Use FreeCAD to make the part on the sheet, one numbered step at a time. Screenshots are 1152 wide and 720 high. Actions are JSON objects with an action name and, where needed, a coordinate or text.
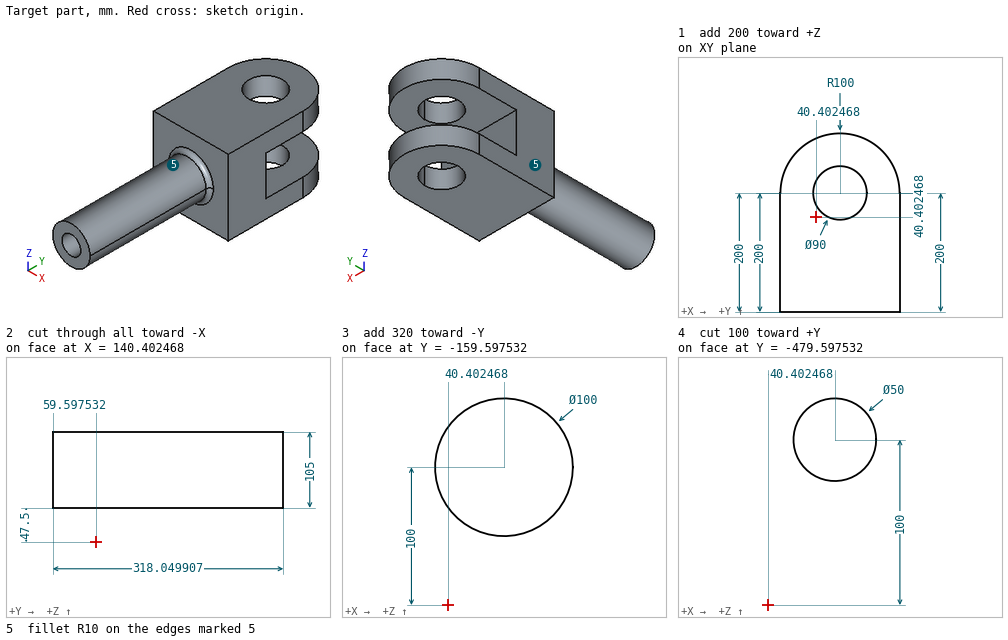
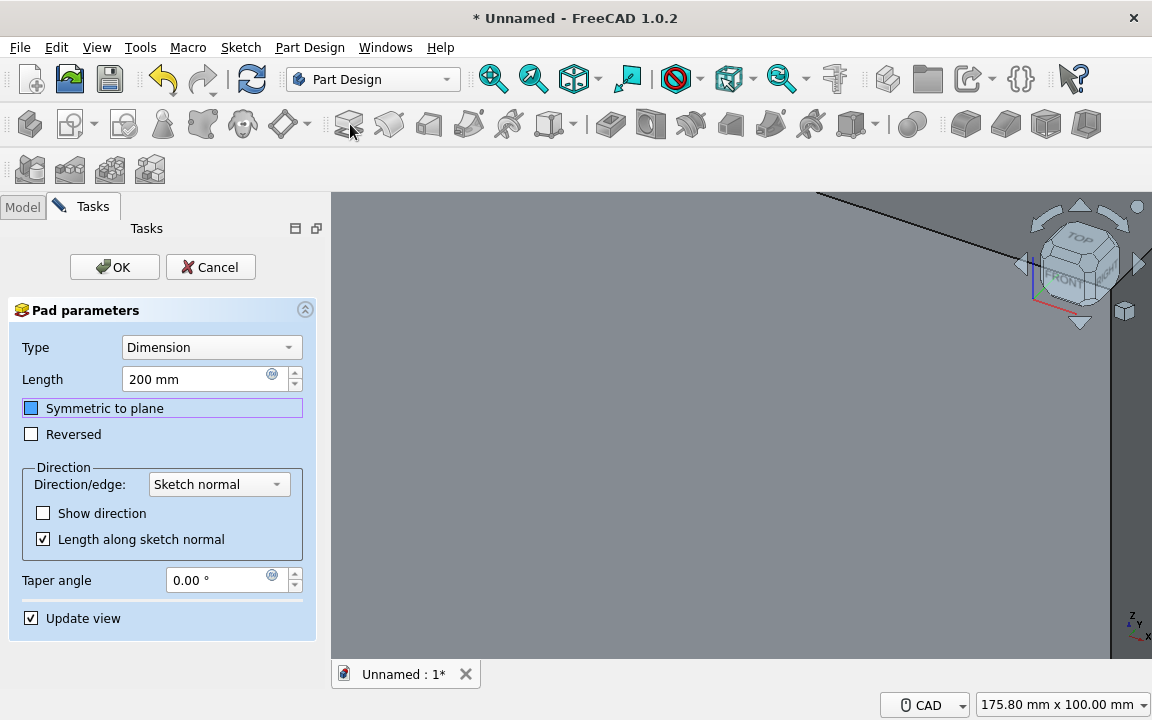
{"action": "left_click", "coordinate": [115, 267]}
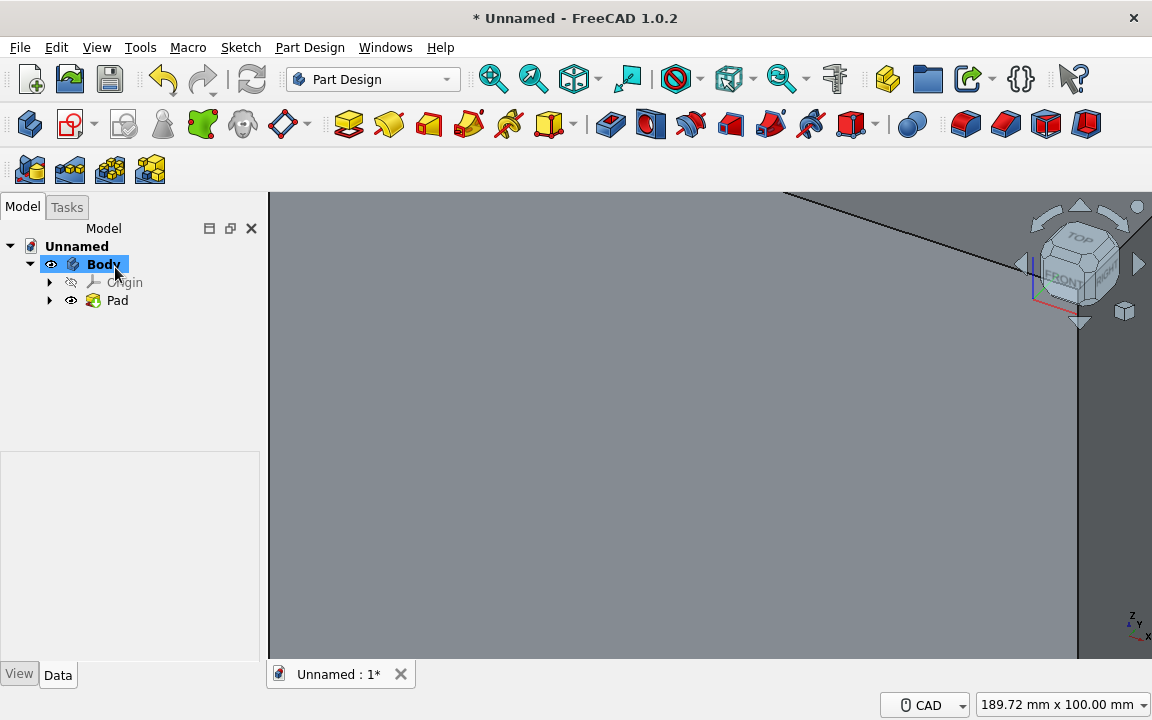
{"action": "key", "text": "v f"}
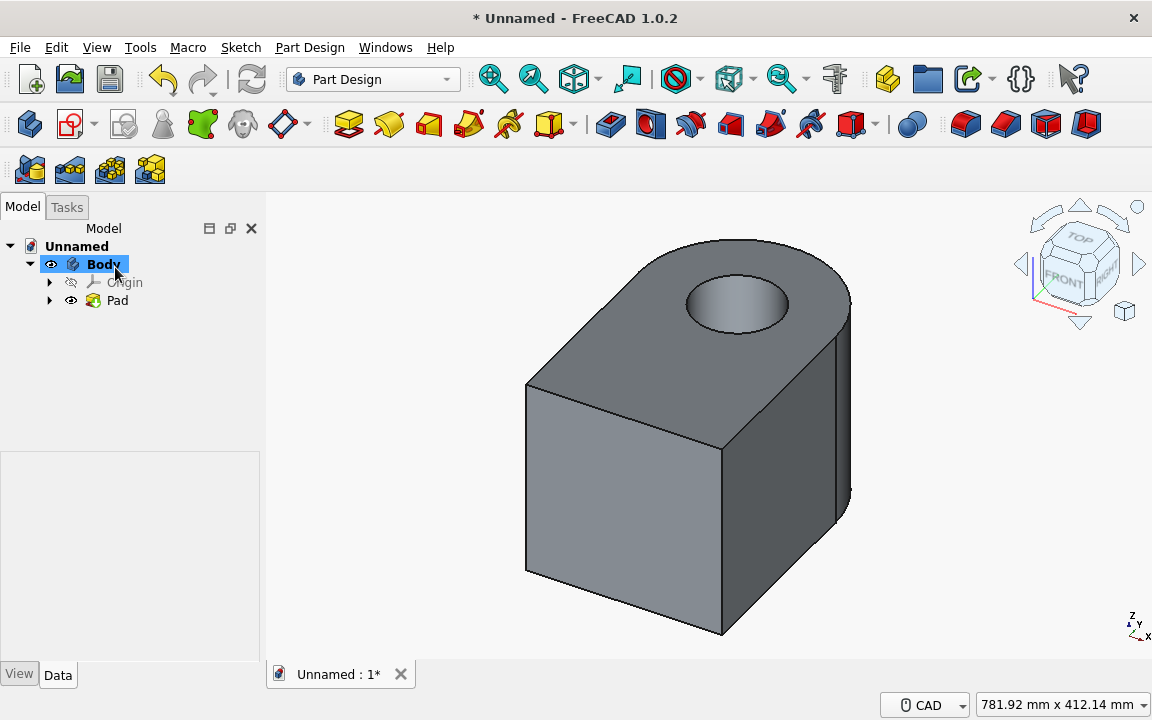
{"action": "left_click", "coordinate": [779, 485]}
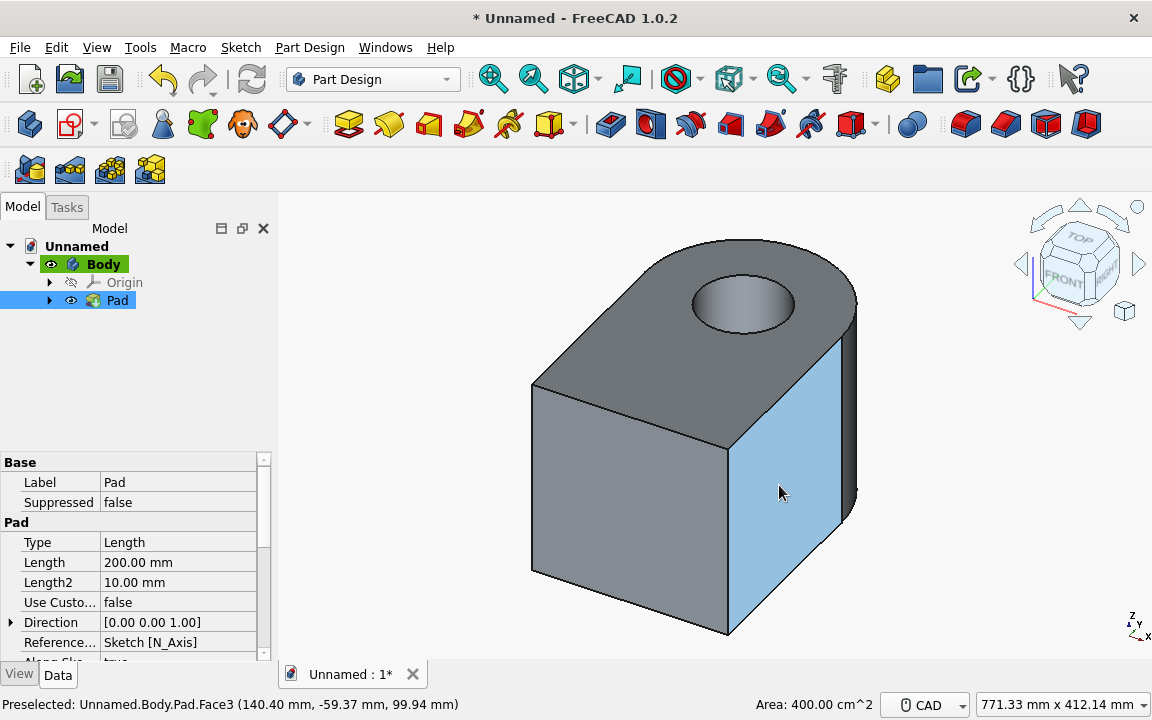
{"action": "left_click", "coordinate": [70, 124]}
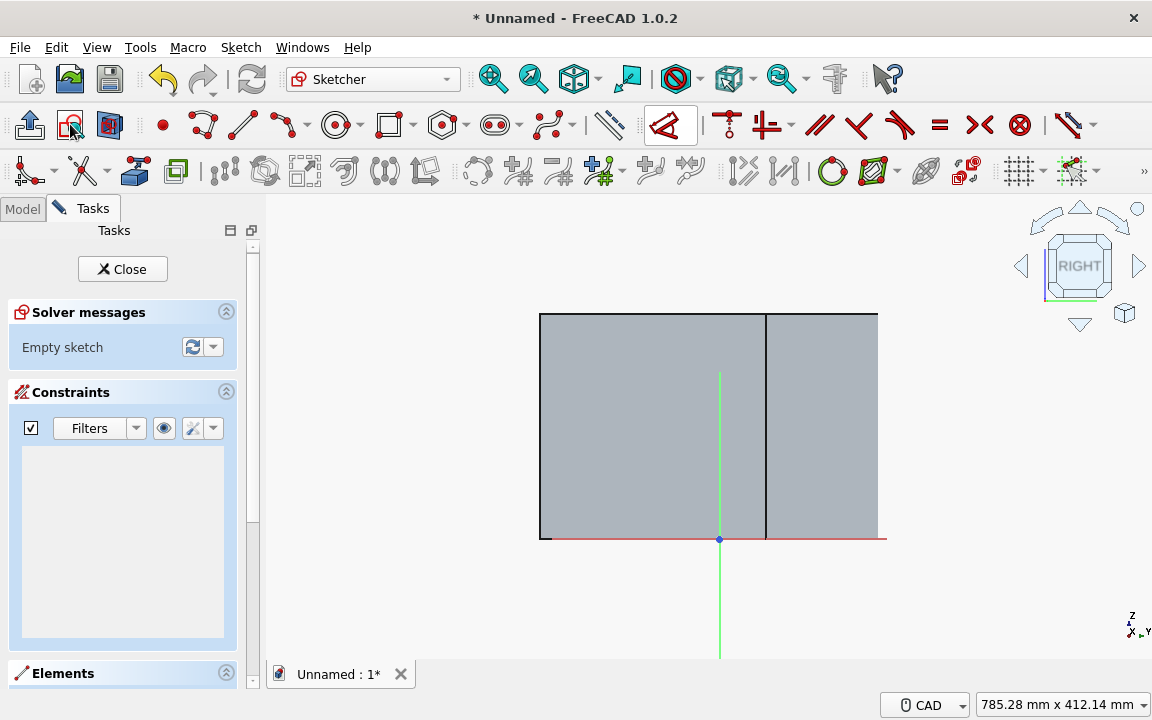
{"action": "scroll", "coordinate": [294, 305], "scroll_direction": "down", "scroll_amount": 1}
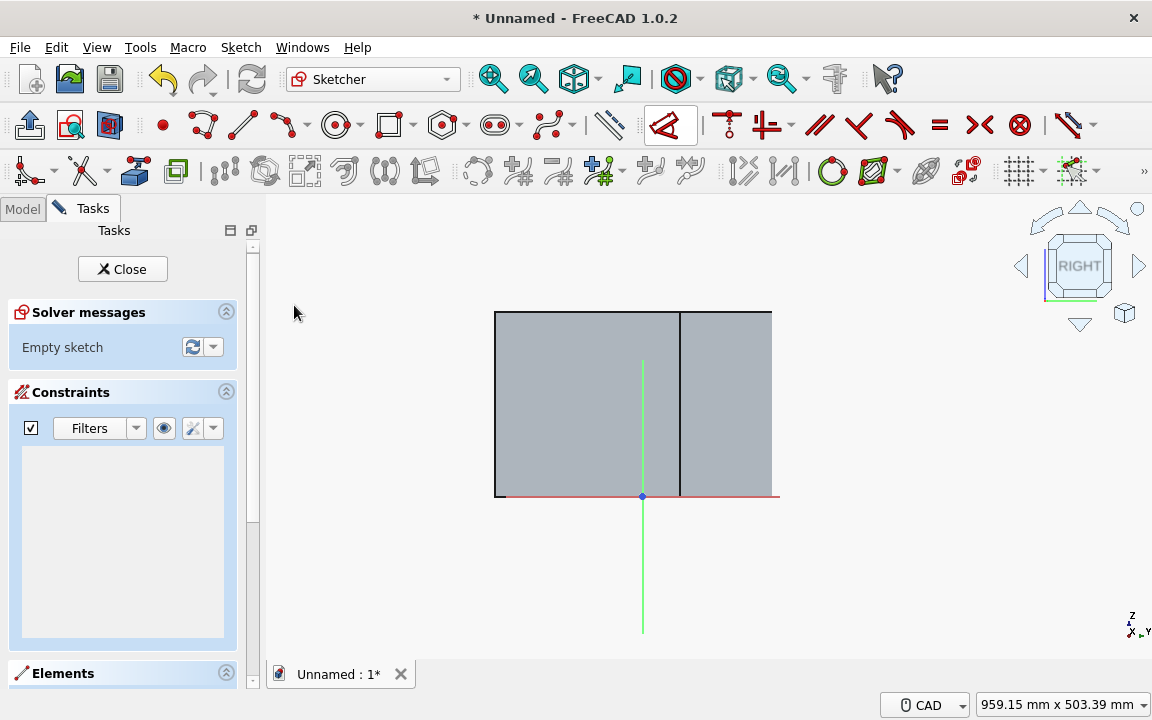
{"action": "scroll", "coordinate": [849, 426], "scroll_direction": "up", "scroll_amount": 3}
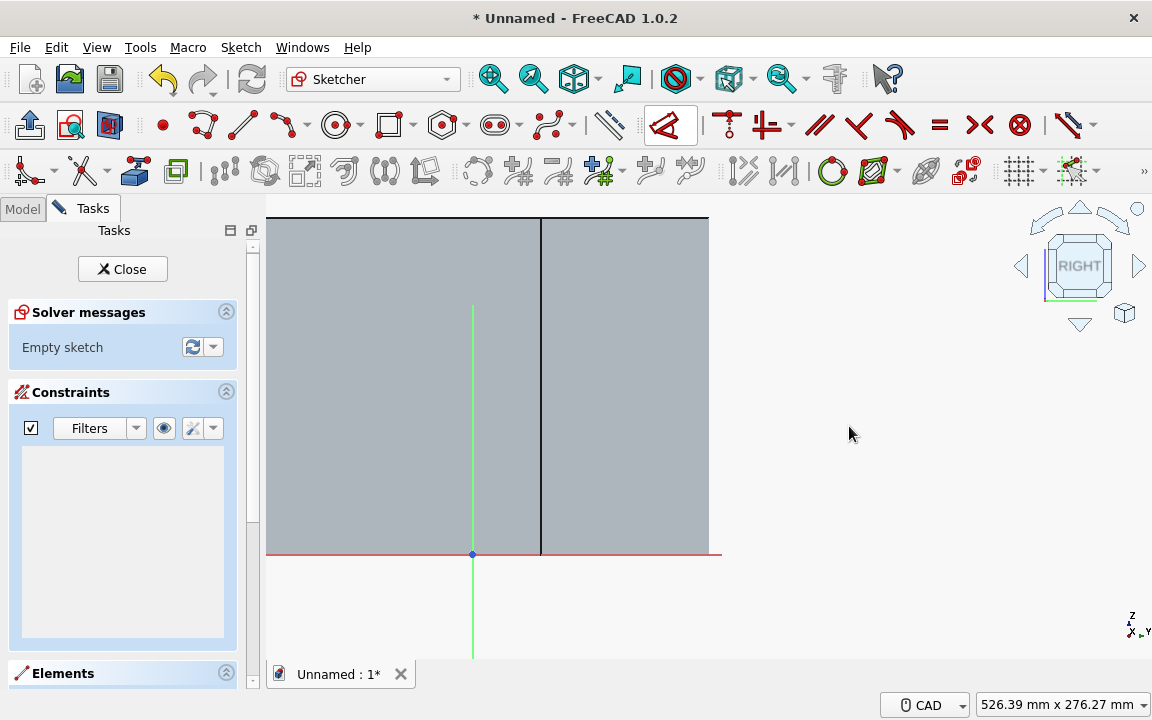
{"action": "left_click", "coordinate": [390, 126]}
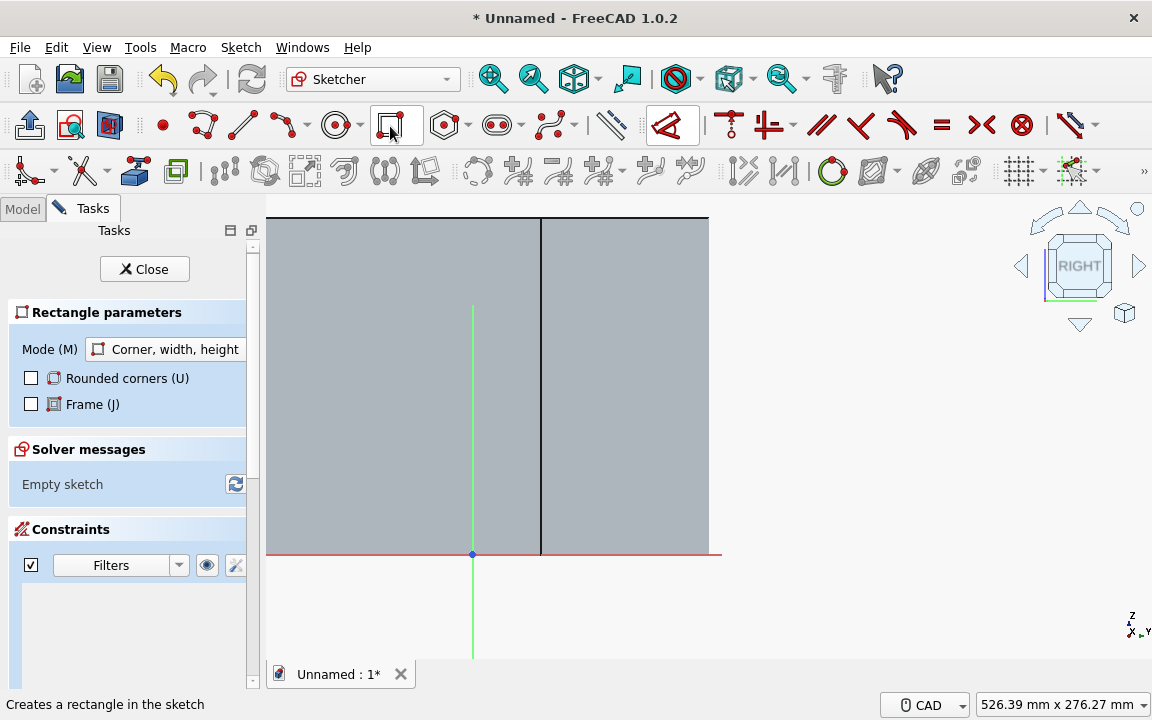
{"action": "left_click", "coordinate": [372, 298]}
{"action": "mouse_move", "coordinate": [908, 475]}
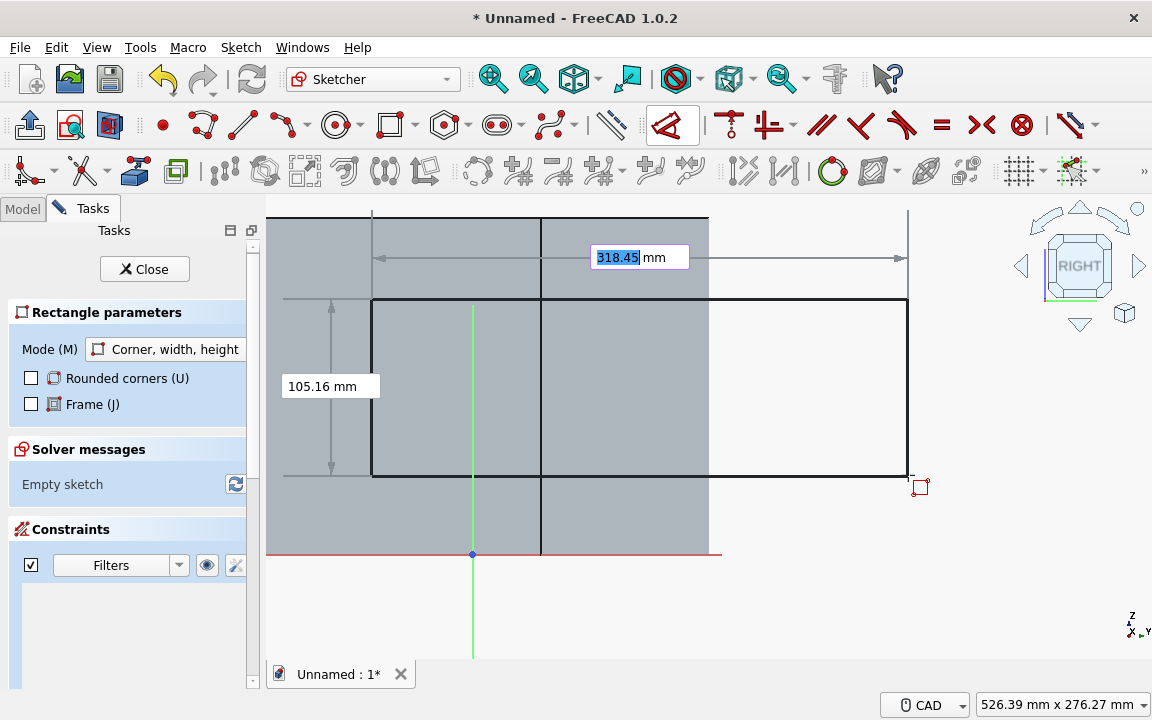
{"action": "type", "text": "318.049907"}
{"action": "key", "text": "Tab"}
{"action": "type", "text": "105"}
{"action": "key", "text": "Return"}
{"action": "key", "text": "Escape"}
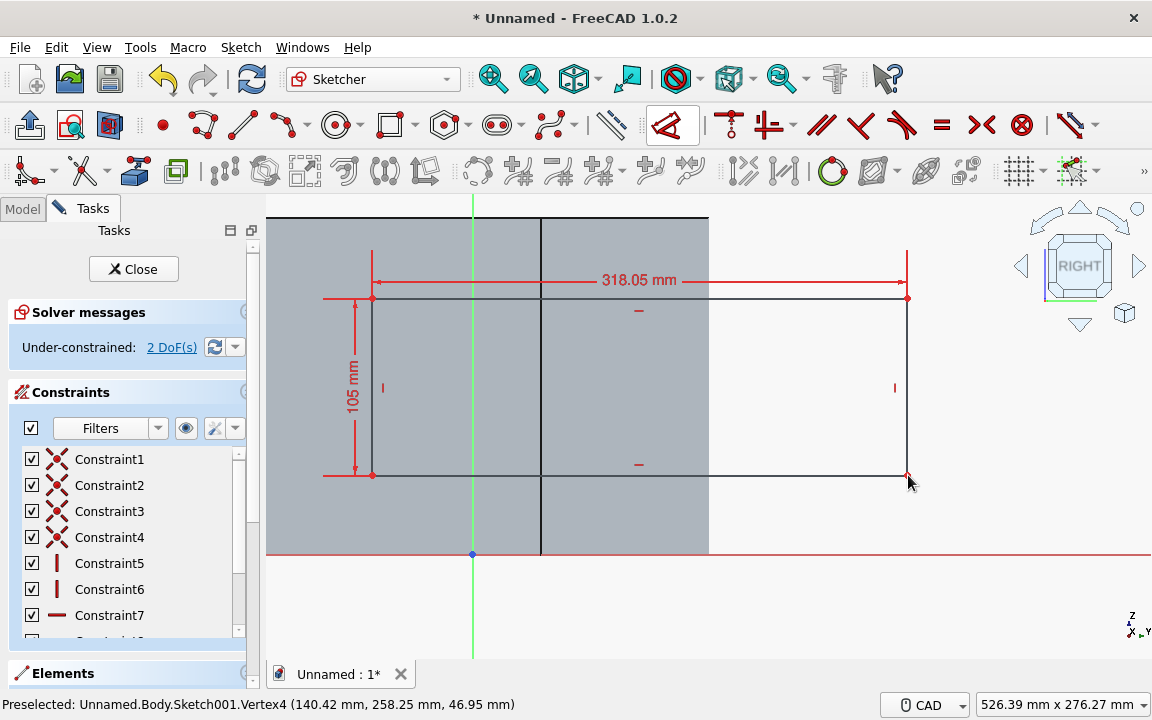
{"action": "left_click", "coordinate": [372, 476]}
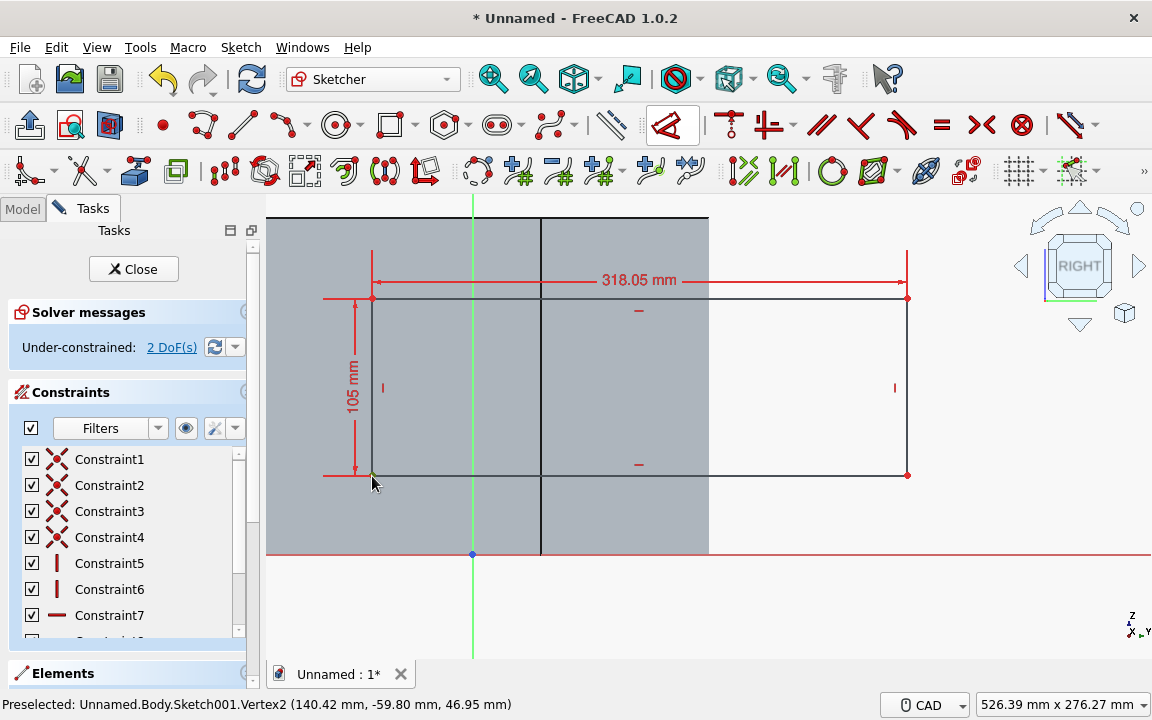
{"action": "key", "text": "i"}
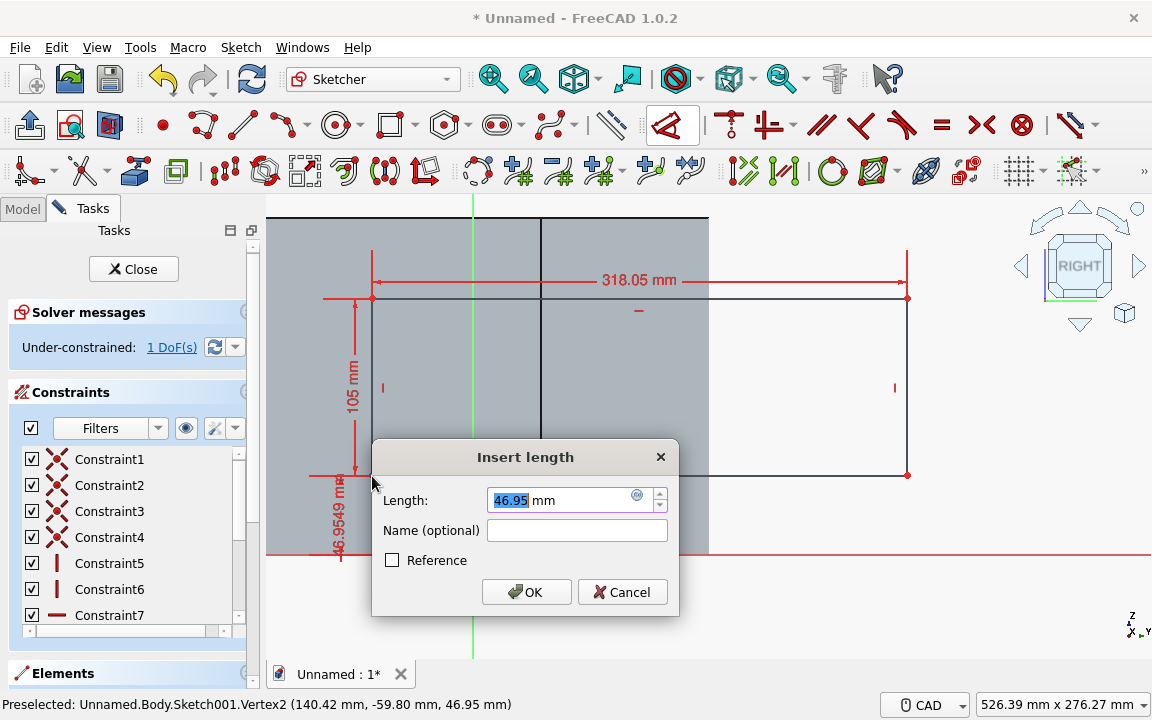
{"action": "type", "text": "47.5"}
{"action": "key", "text": "Return"}